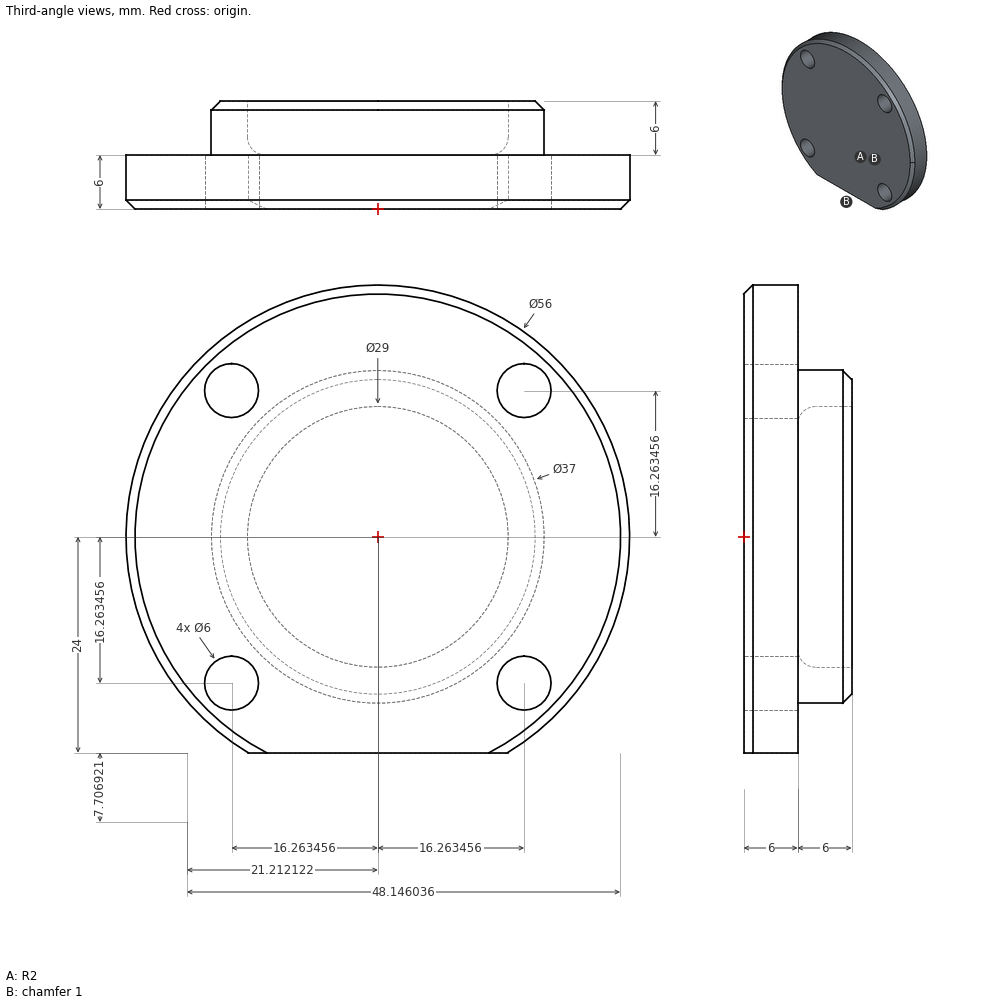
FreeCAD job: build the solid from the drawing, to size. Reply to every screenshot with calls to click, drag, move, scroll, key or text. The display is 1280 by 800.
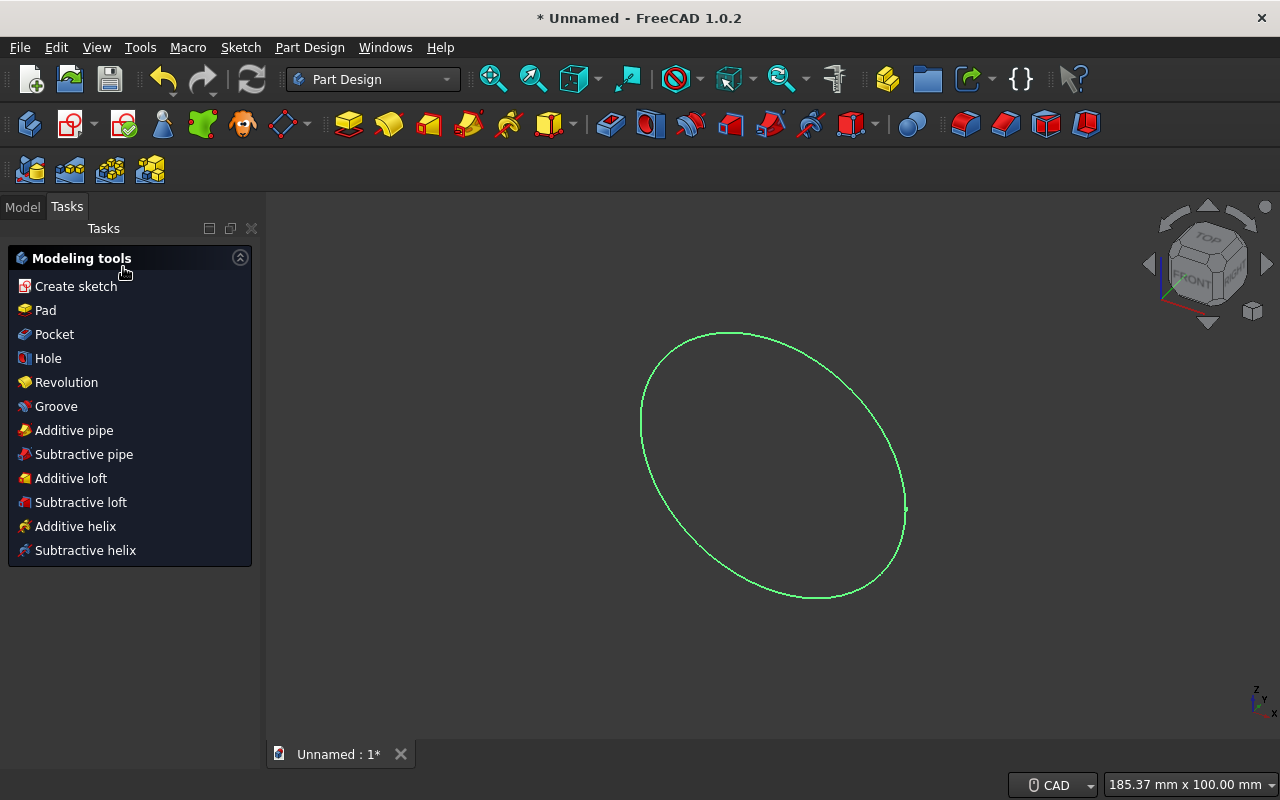
click(350, 124)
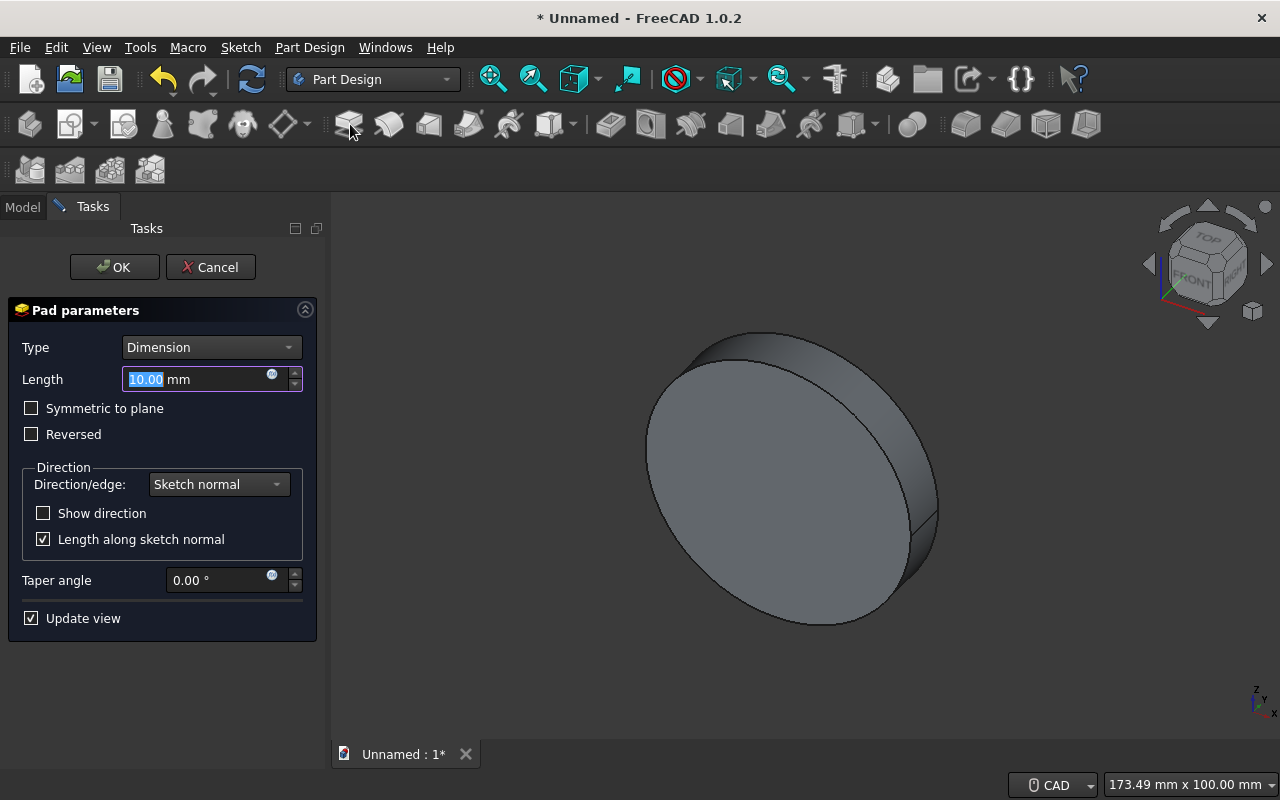
text(6)
key(Tab)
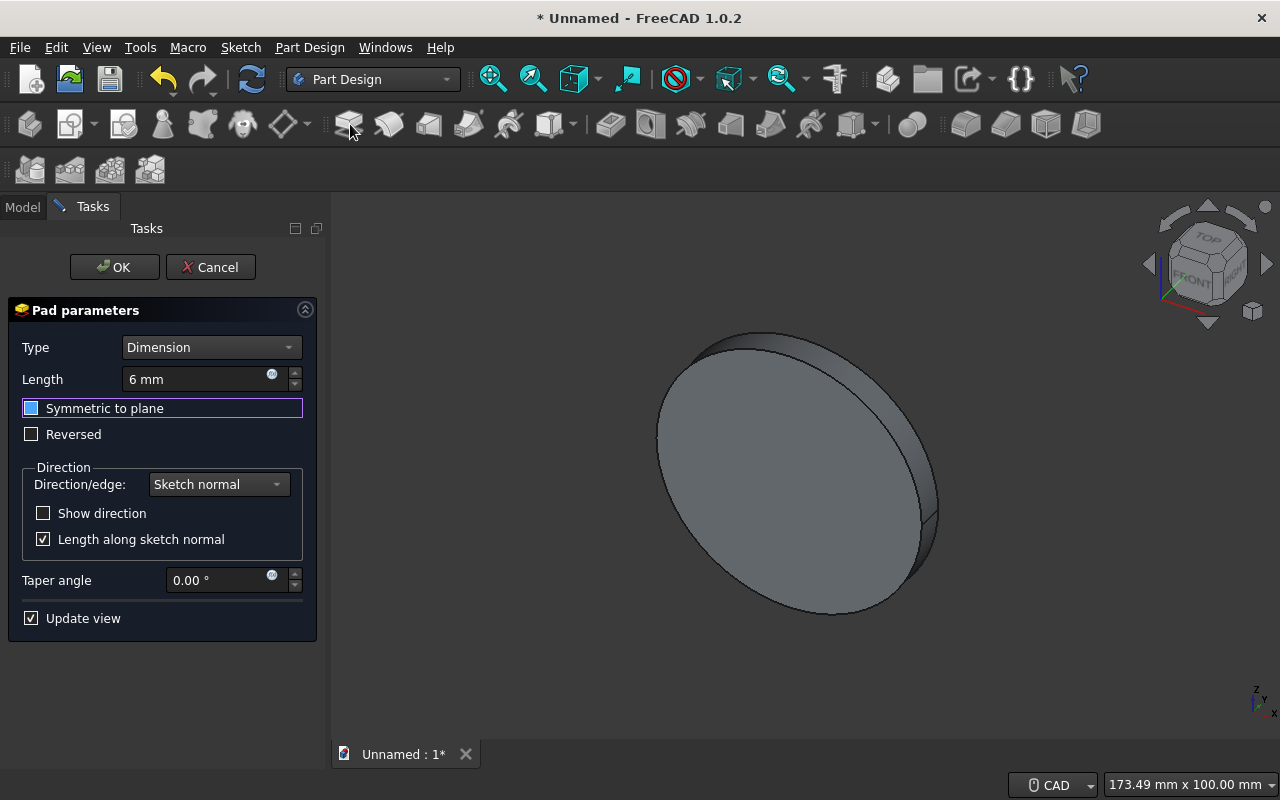
click(30, 434)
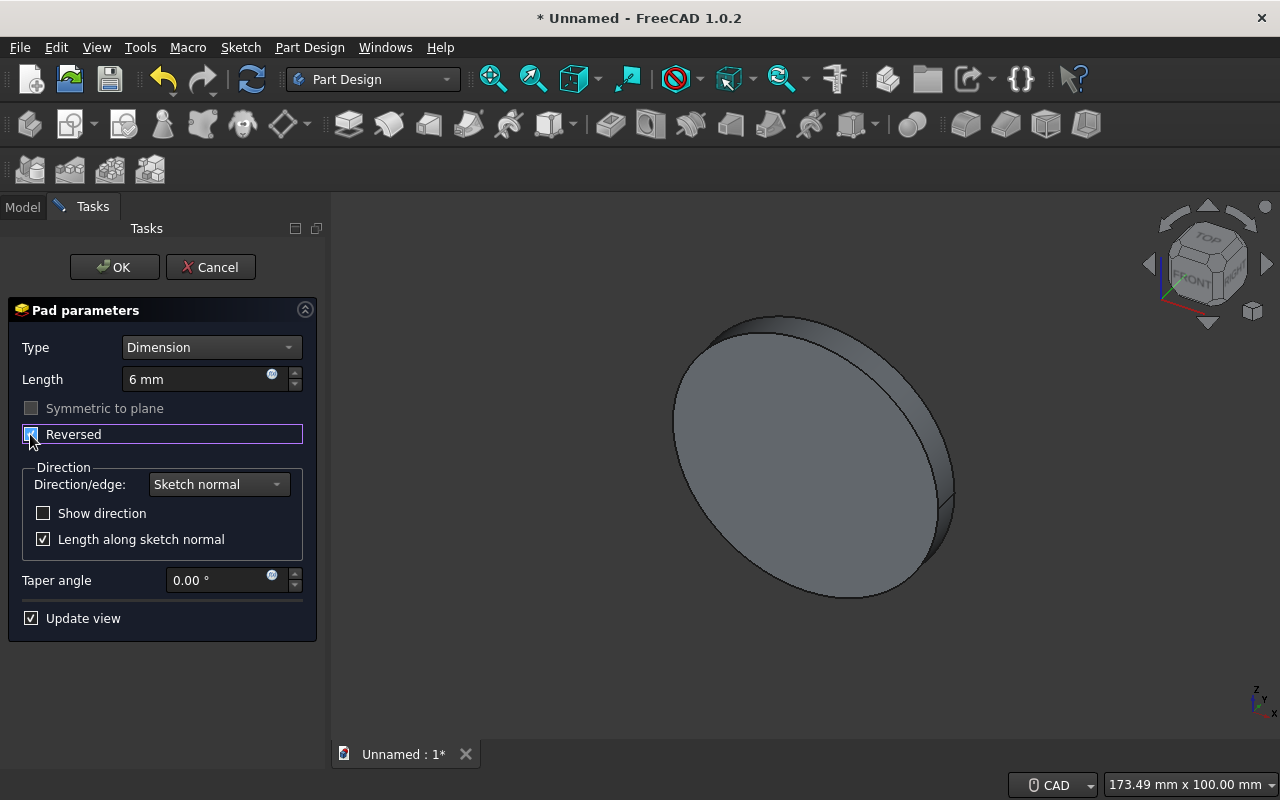
click(115, 267)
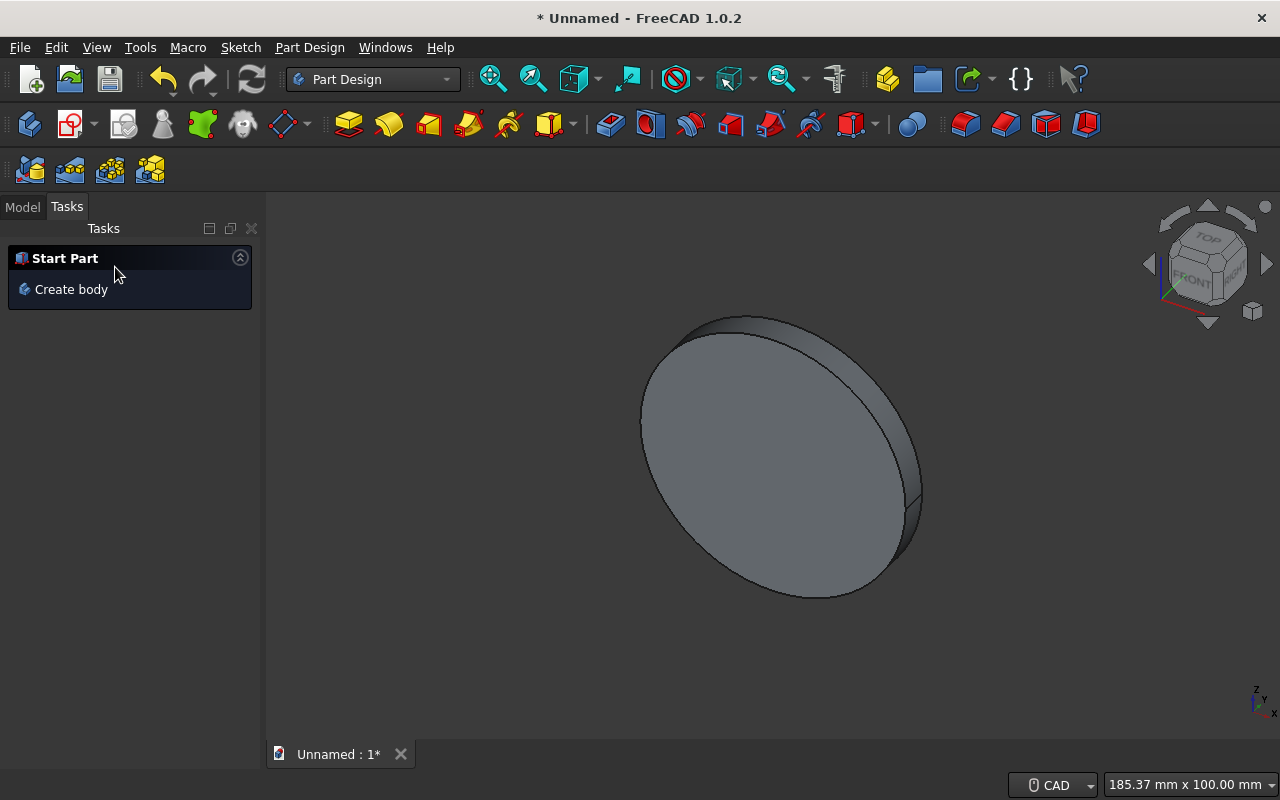
key(4)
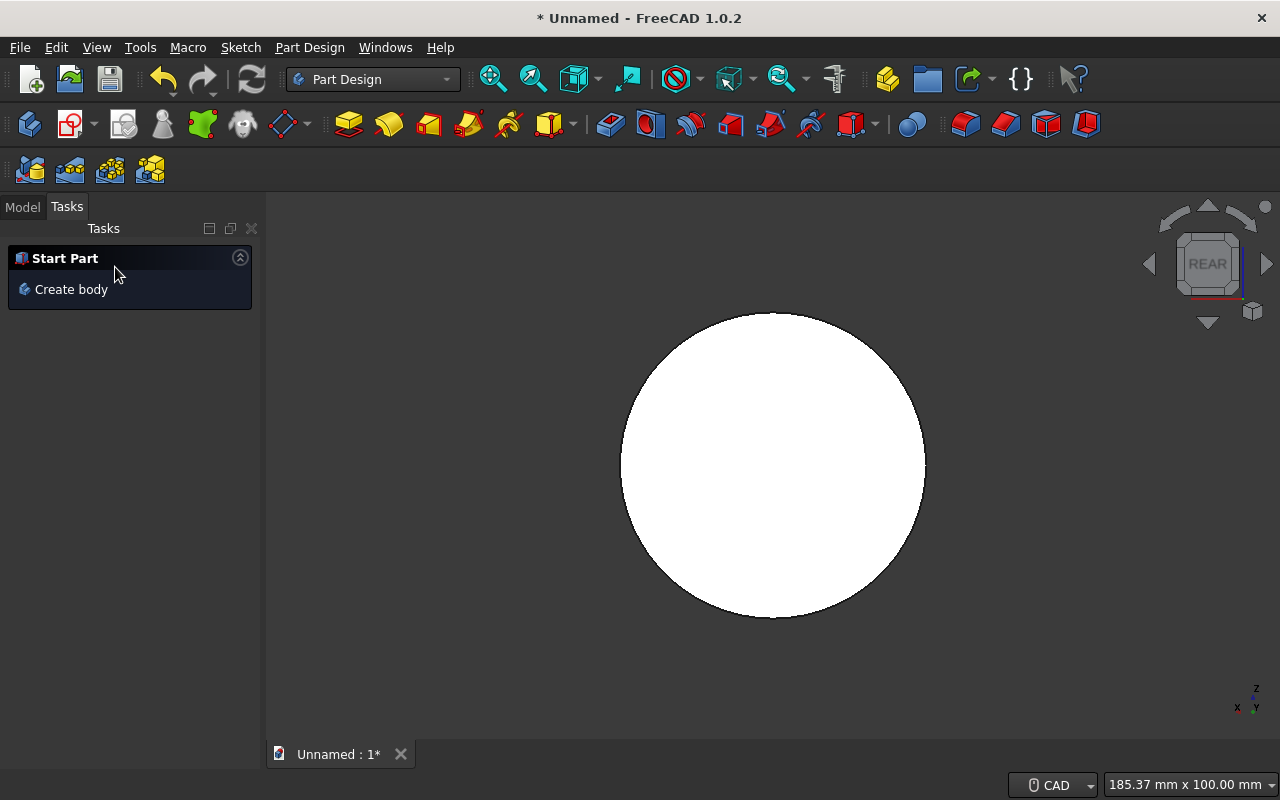
click(773, 464)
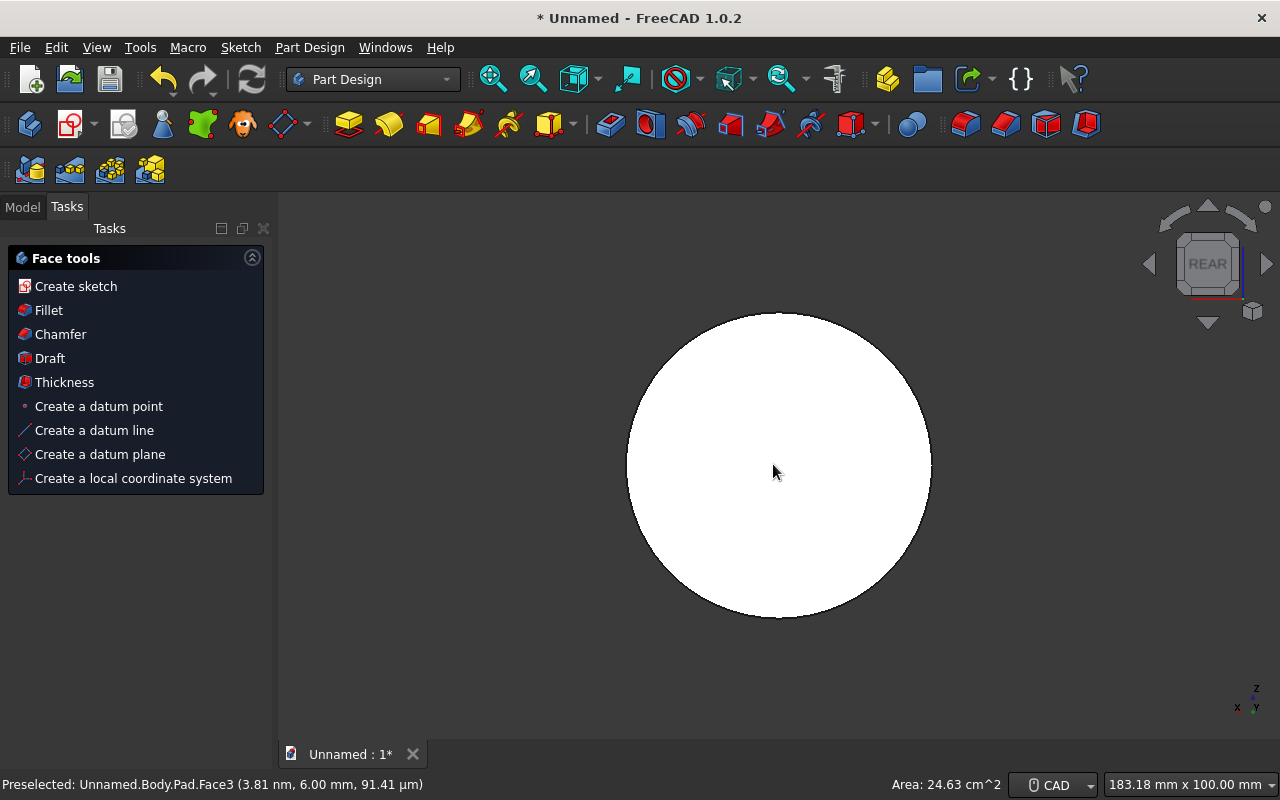
click(70, 124)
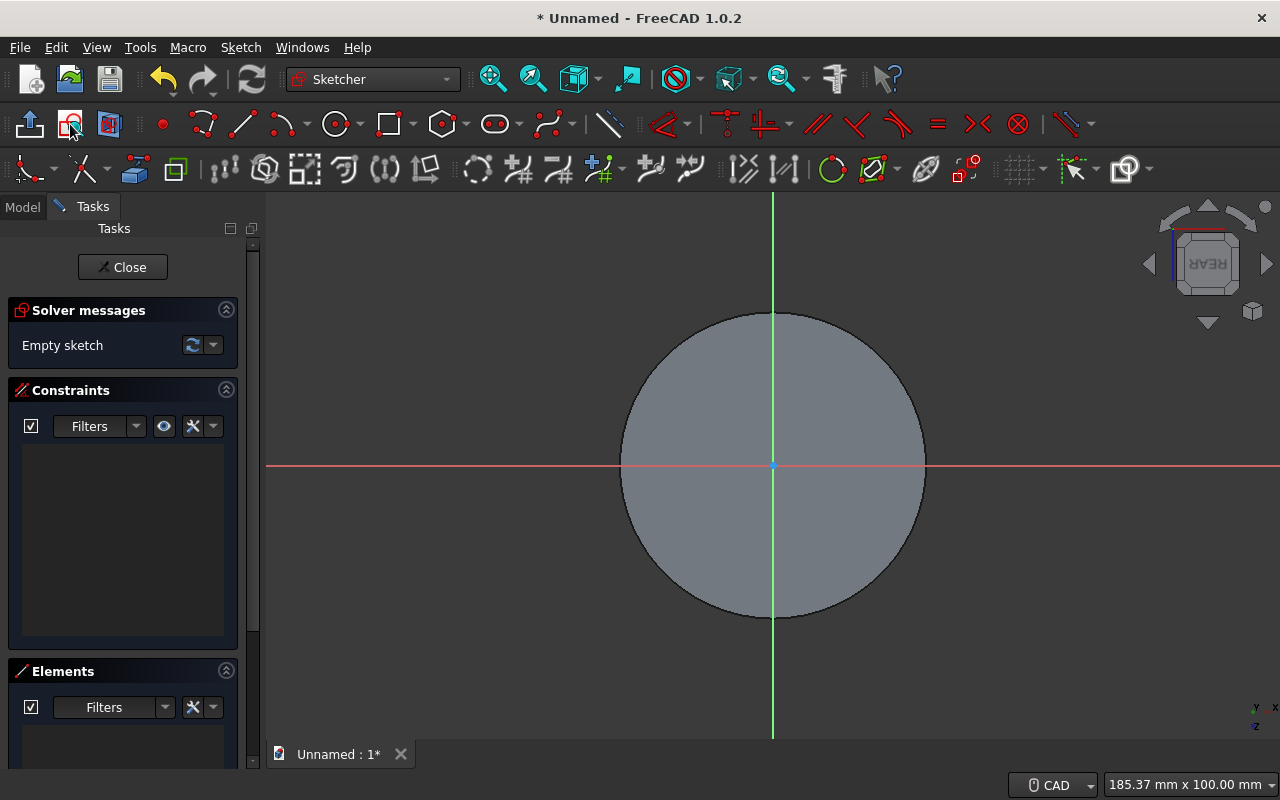
scroll(856, 466, up, 3)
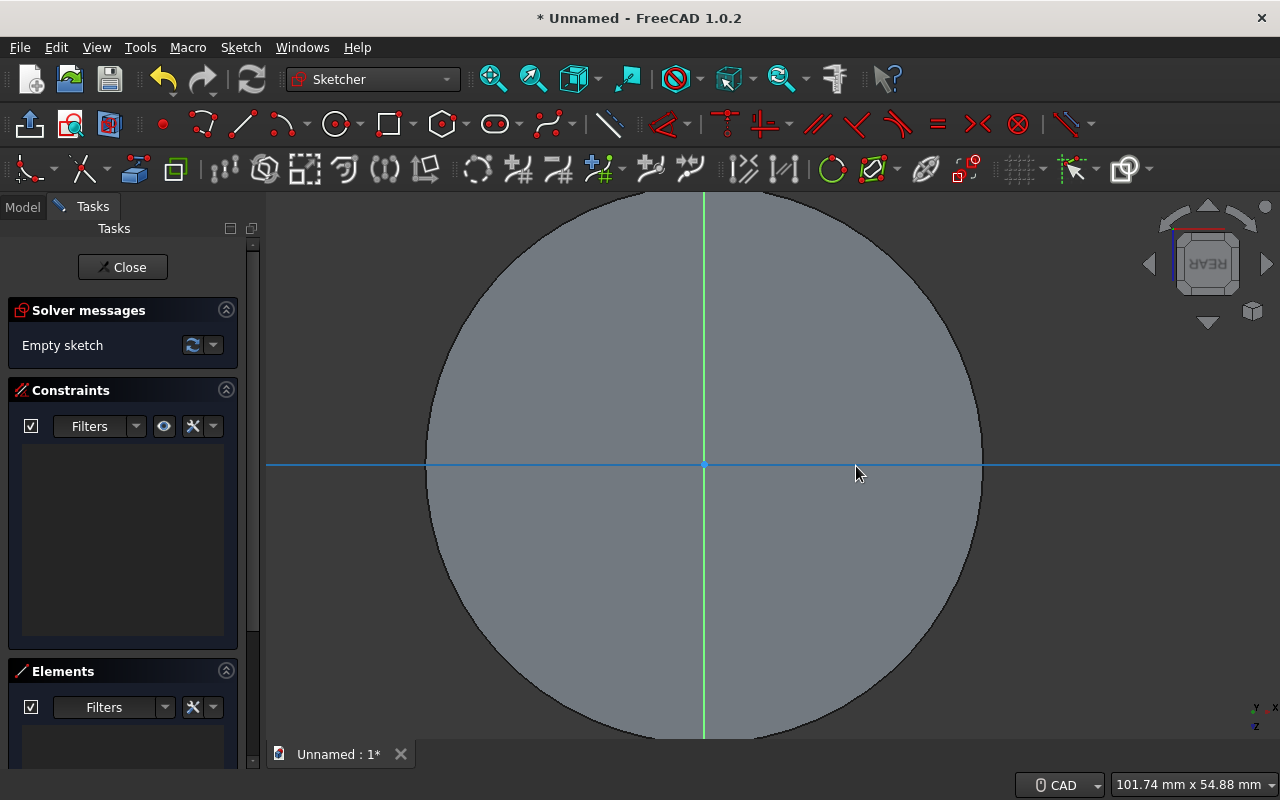
key(g)
key(c)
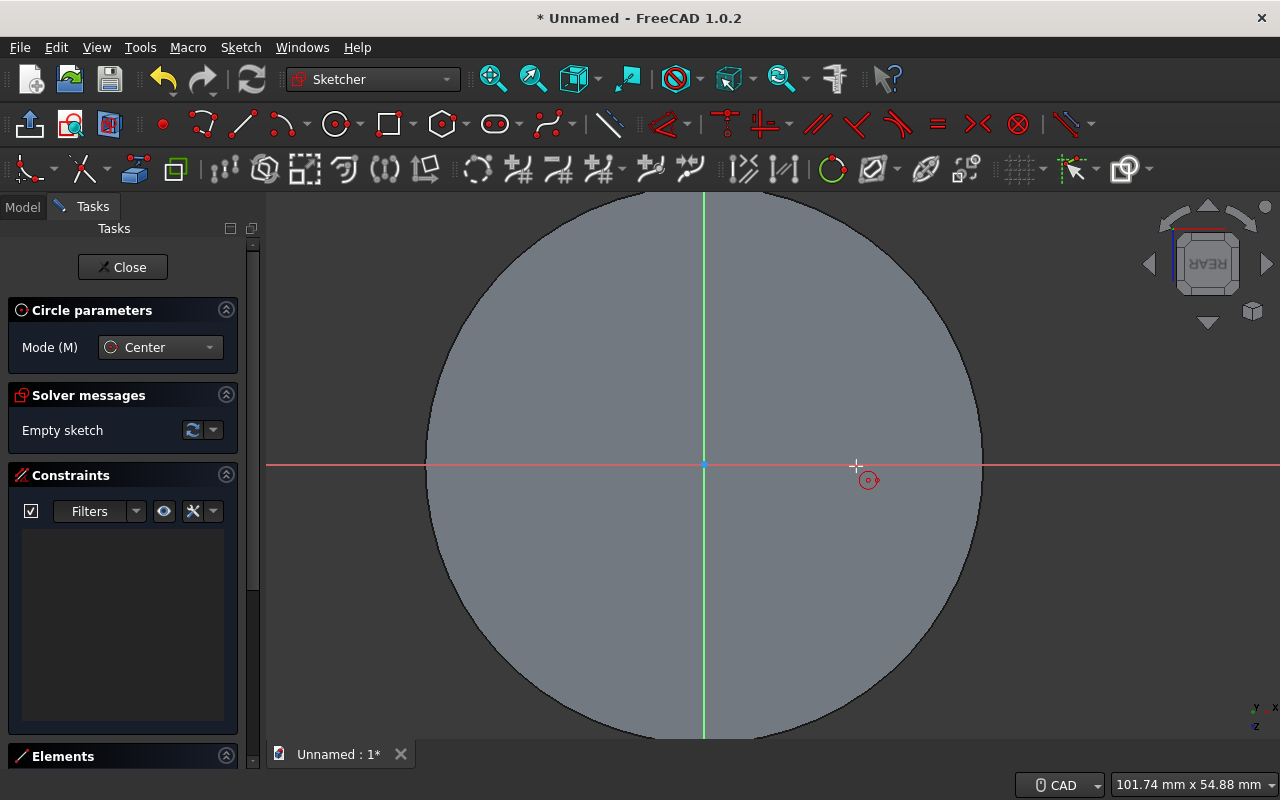
click(704, 465)
click(835, 334)
key(Escape)